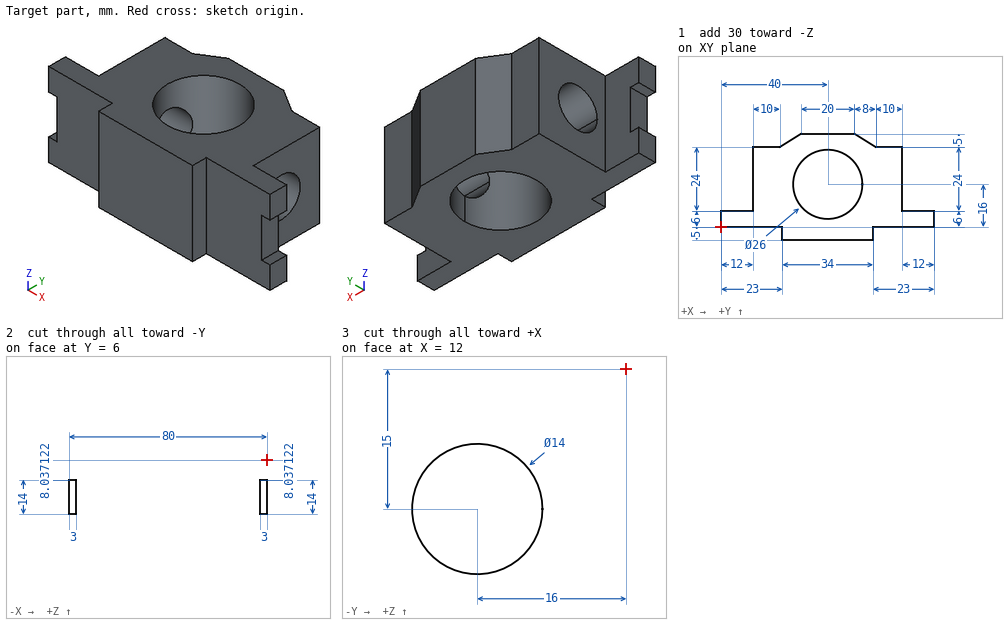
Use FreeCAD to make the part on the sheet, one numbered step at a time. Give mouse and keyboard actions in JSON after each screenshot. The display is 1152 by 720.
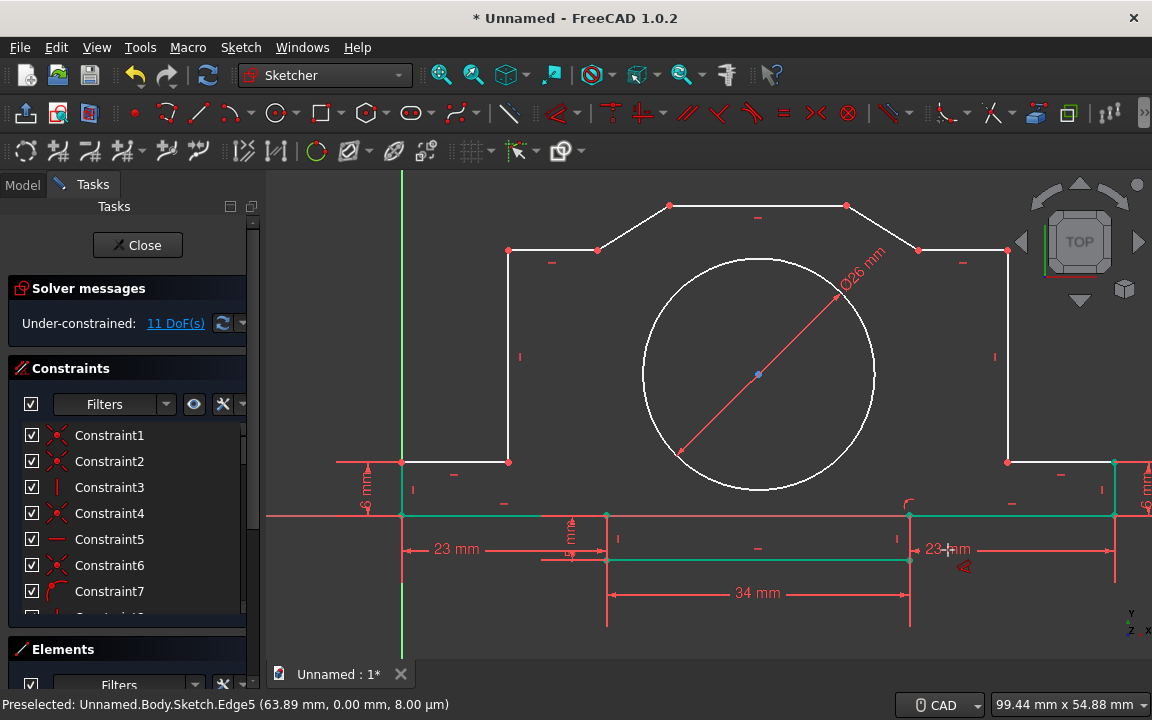
{"action": "scroll", "coordinate": [401, 480], "scroll_direction": "down", "scroll_amount": 2}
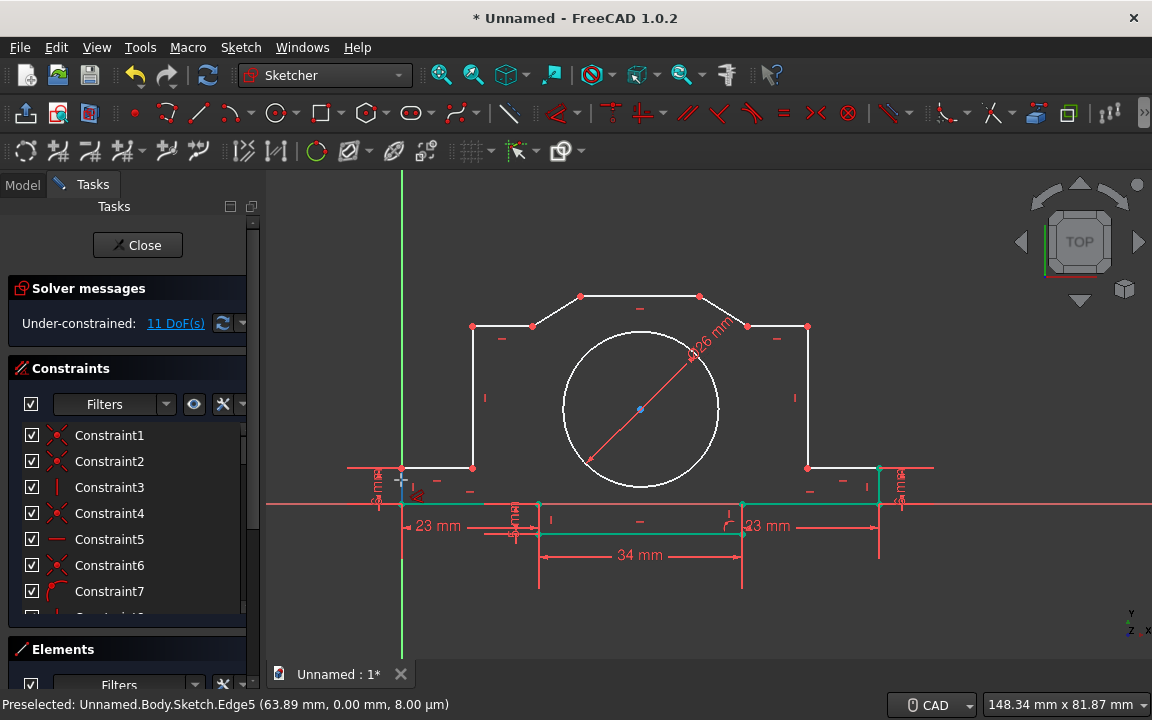
{"action": "left_click", "coordinate": [858, 468]}
{"action": "left_click", "coordinate": [844, 434]}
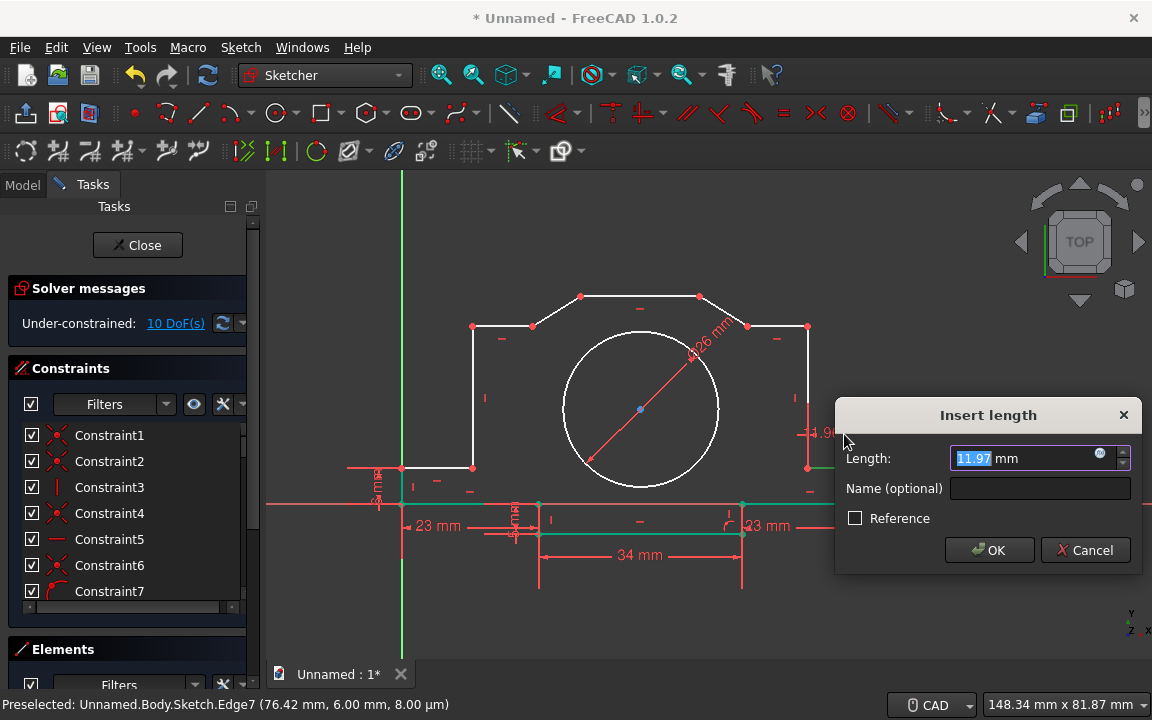
{"action": "type", "text": "12"}
{"action": "key", "text": "Return"}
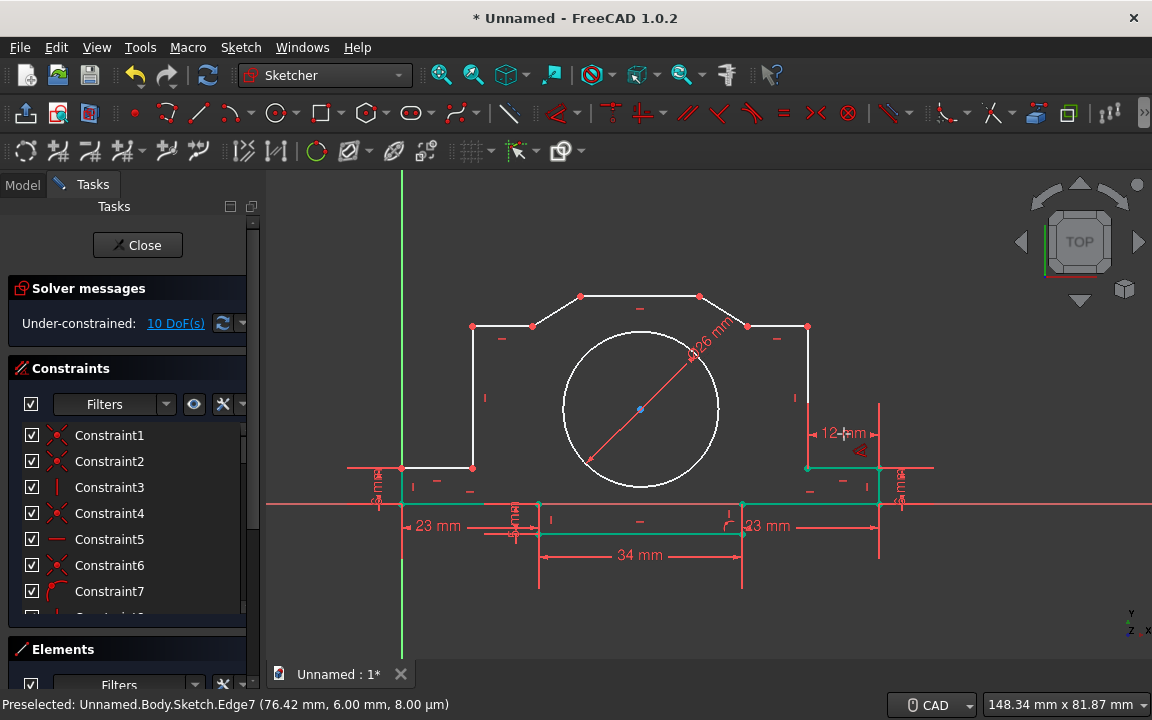
{"action": "left_click", "coordinate": [808, 426]}
{"action": "left_click", "coordinate": [842, 397]}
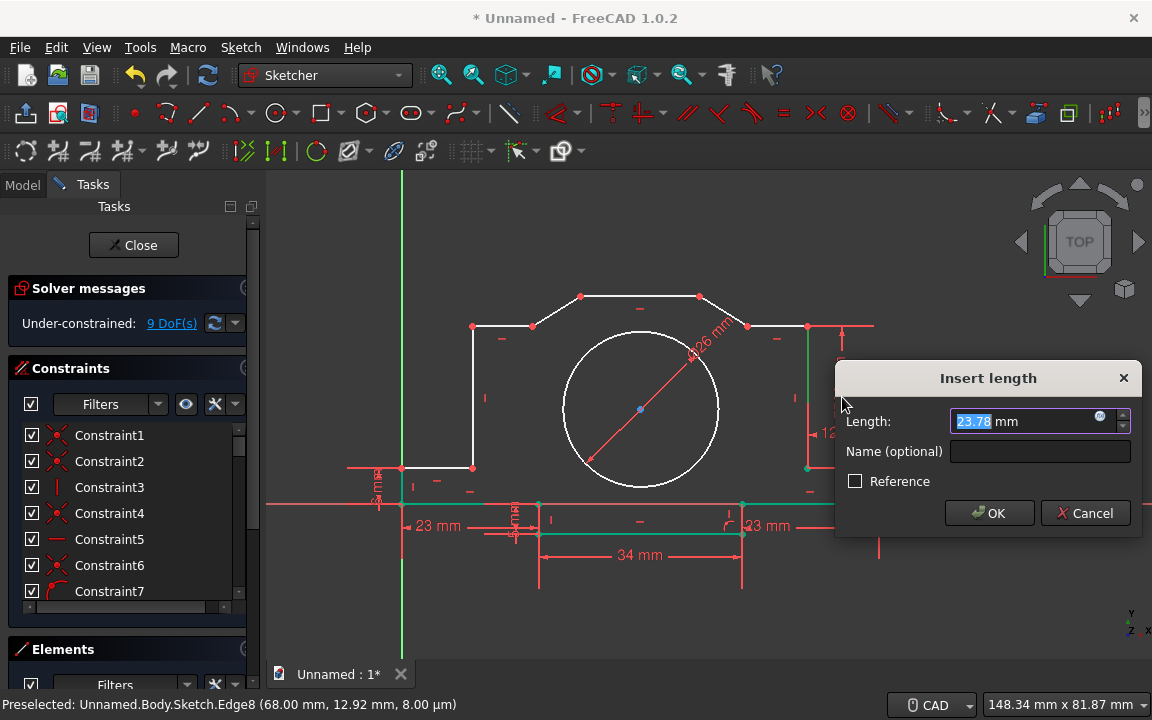
{"action": "type", "text": "24"}
{"action": "key", "text": "Return"}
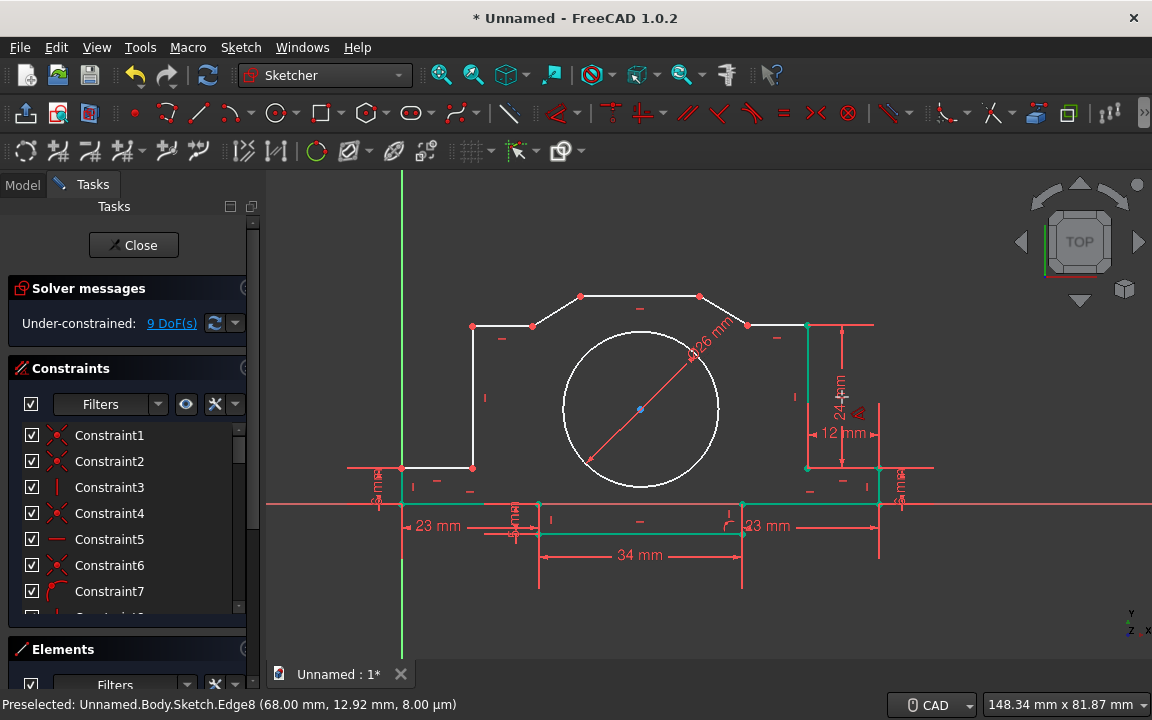
{"action": "left_click", "coordinate": [790, 325]}
{"action": "left_click", "coordinate": [778, 291]}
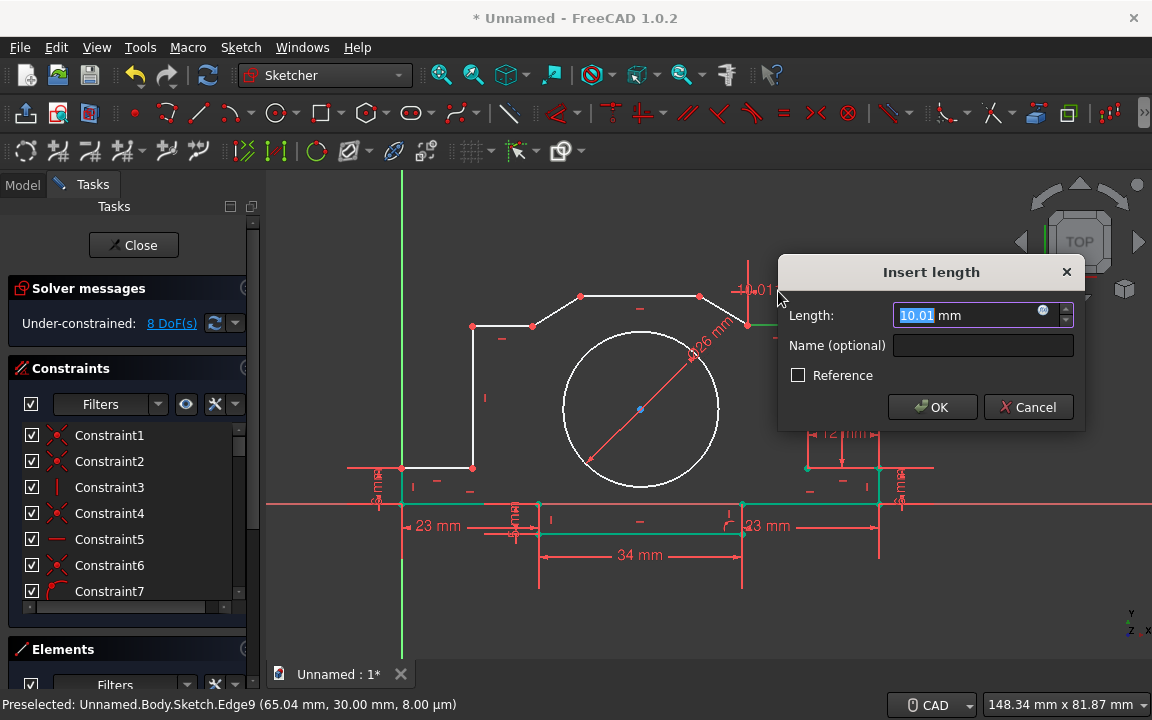
{"action": "type", "text": "10"}
{"action": "key", "text": "Return"}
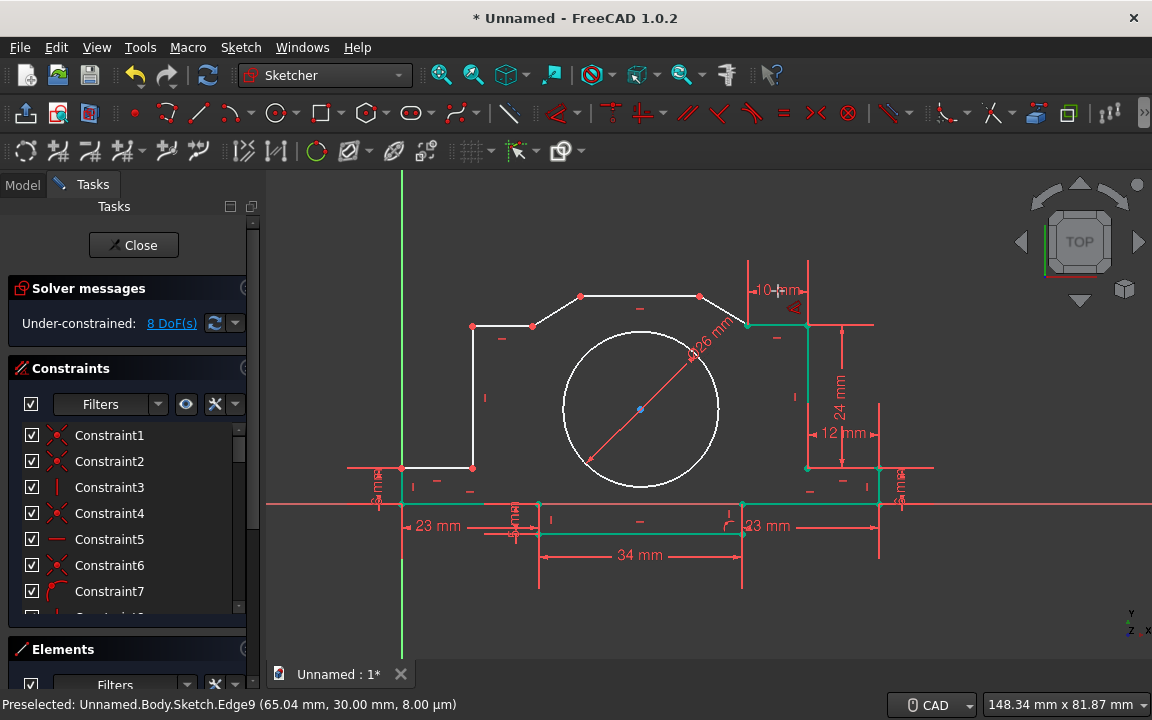
{"action": "left_click", "coordinate": [664, 296]}
{"action": "left_click", "coordinate": [640, 262]}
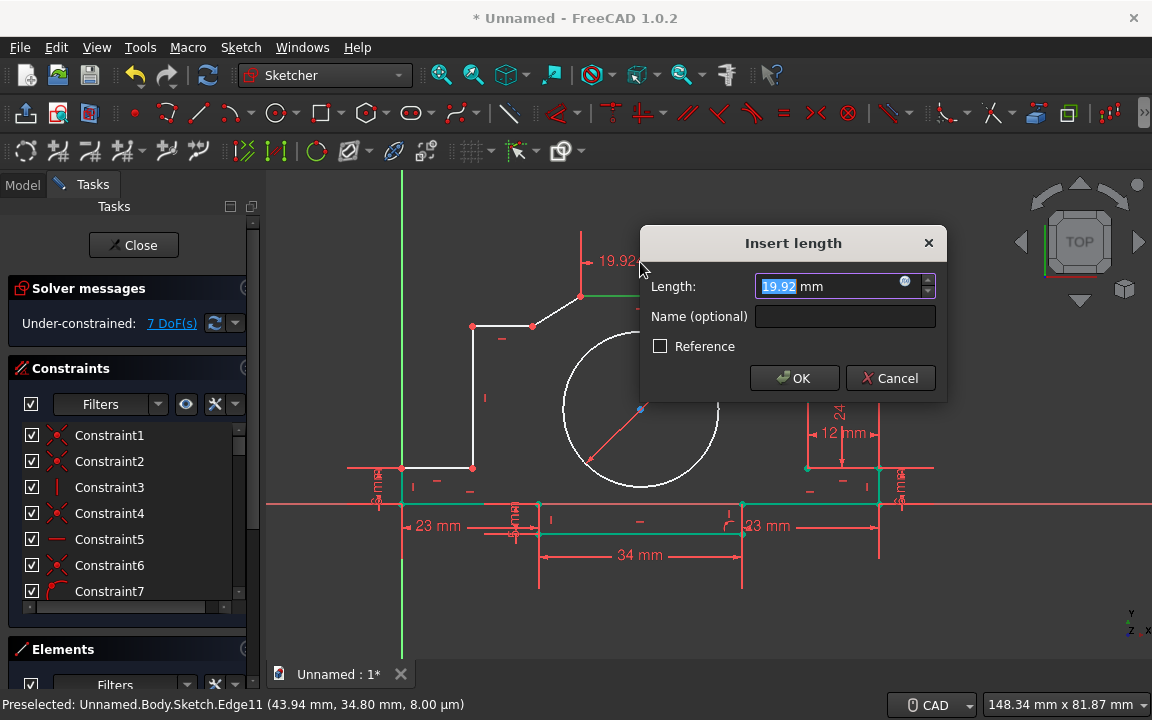
{"action": "type", "text": "20"}
{"action": "key", "text": "Return"}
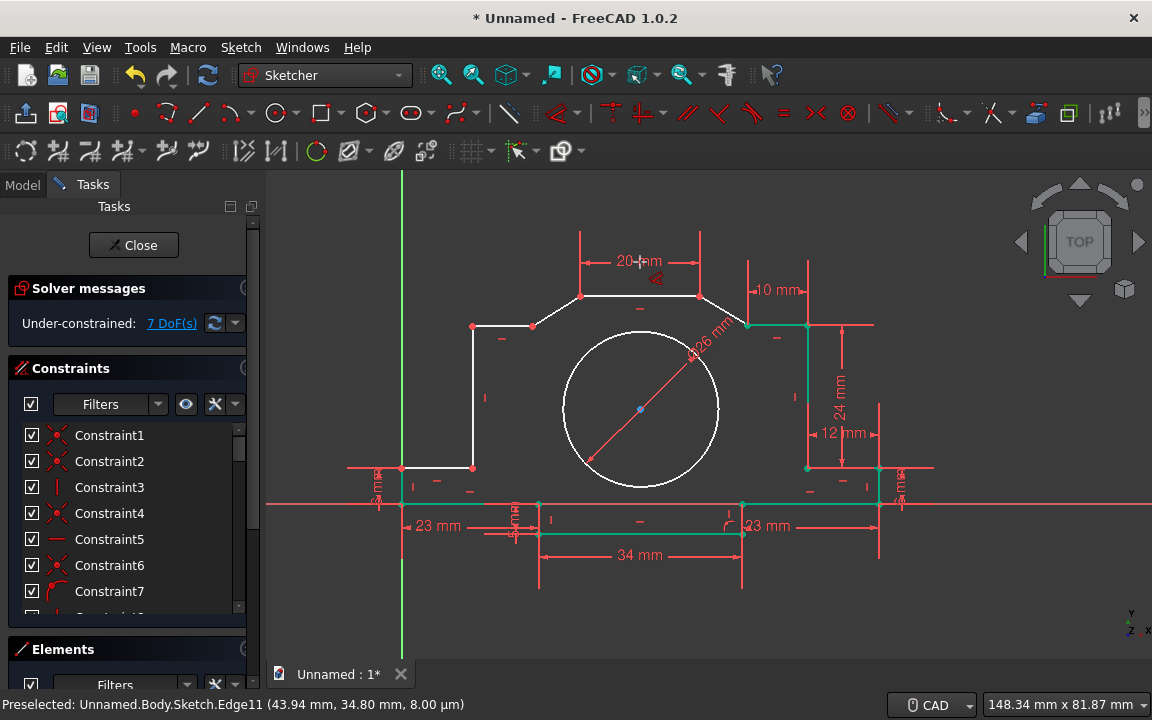
{"action": "left_click", "coordinate": [515, 326]}
{"action": "left_click", "coordinate": [503, 292]}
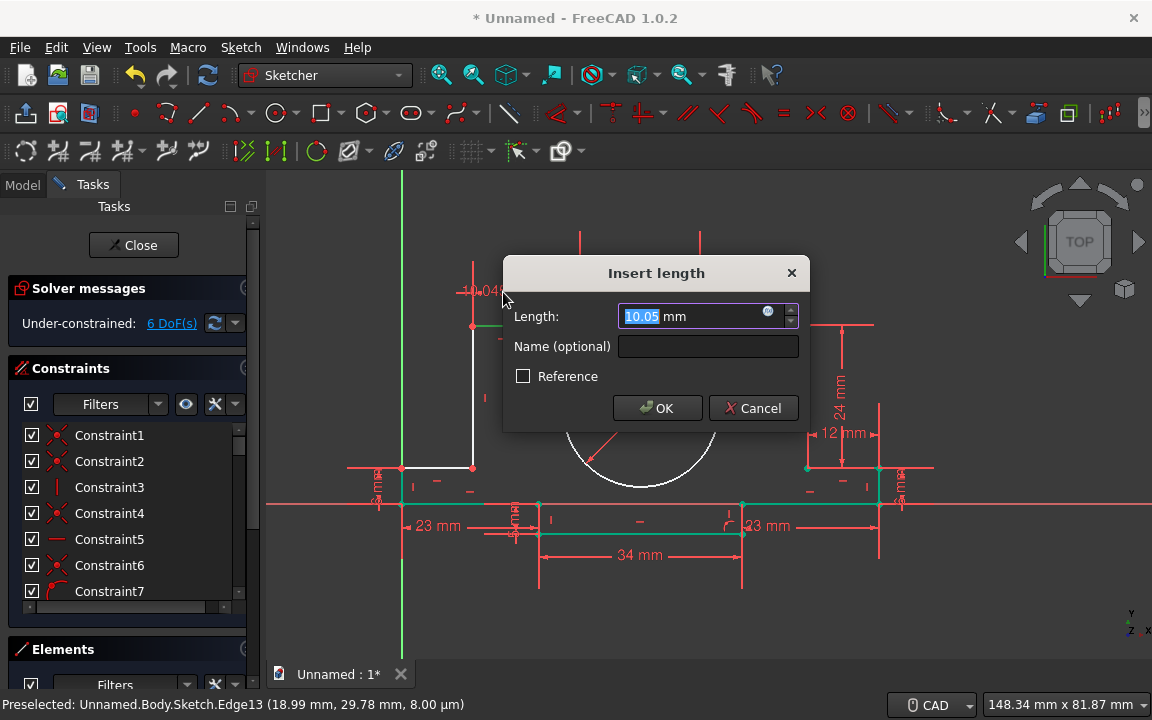
{"action": "type", "text": "10"}
{"action": "key", "text": "Return"}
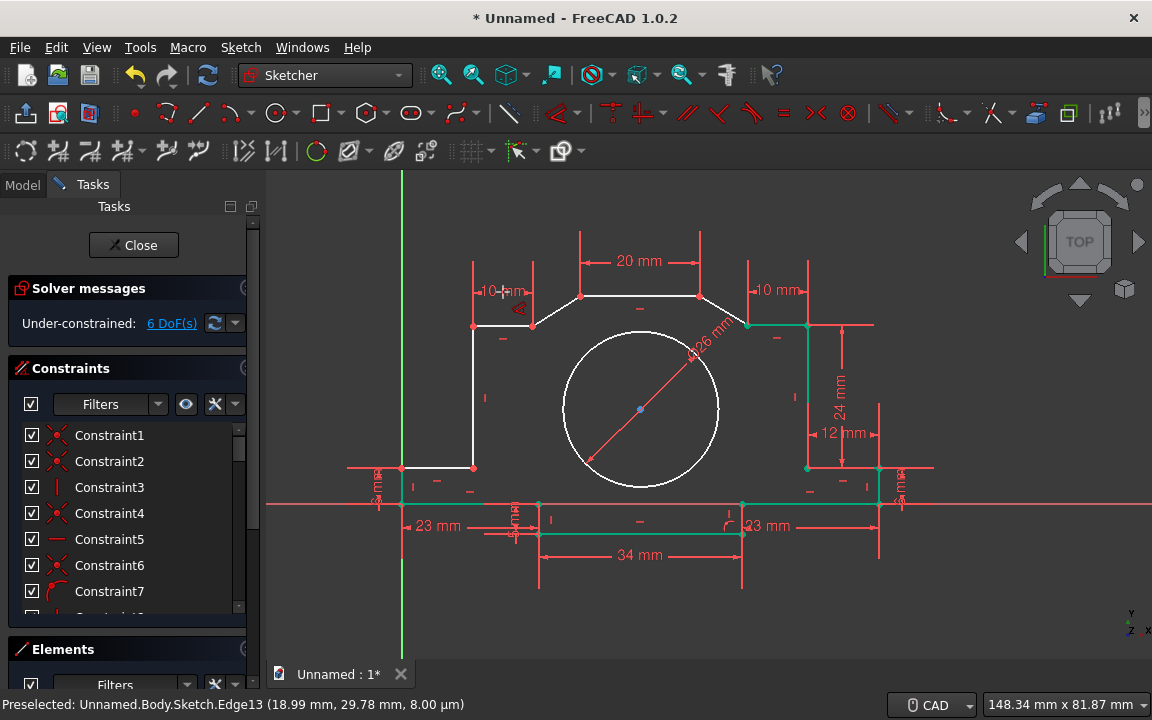
{"action": "left_click", "coordinate": [473, 369]}
{"action": "left_click", "coordinate": [439, 397]}